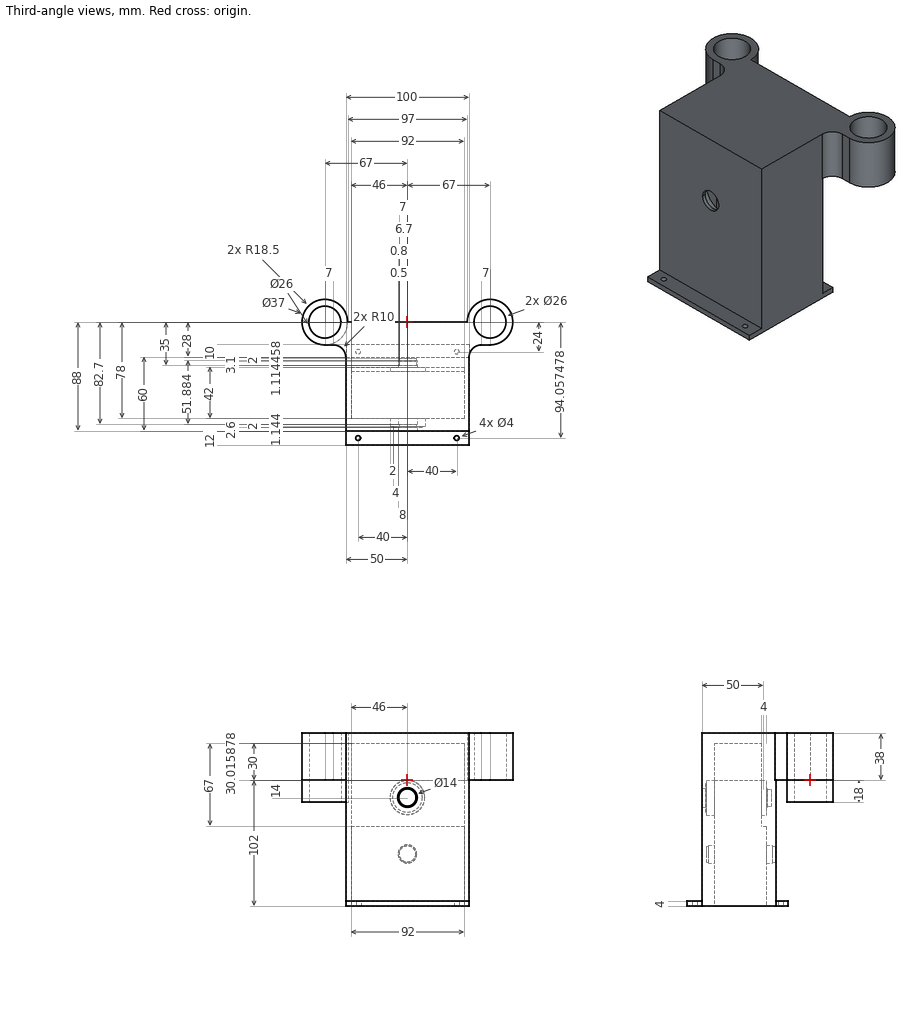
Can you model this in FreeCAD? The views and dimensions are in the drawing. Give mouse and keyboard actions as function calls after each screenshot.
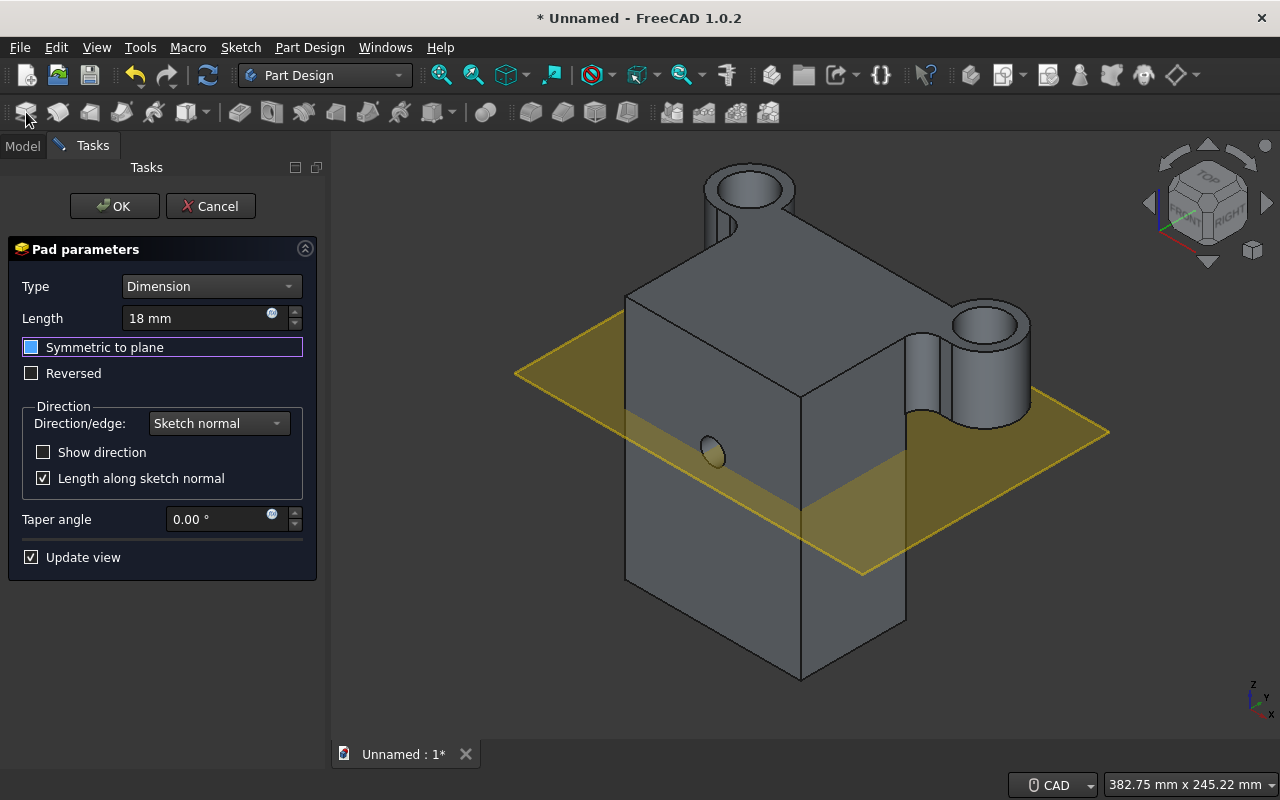
click(115, 206)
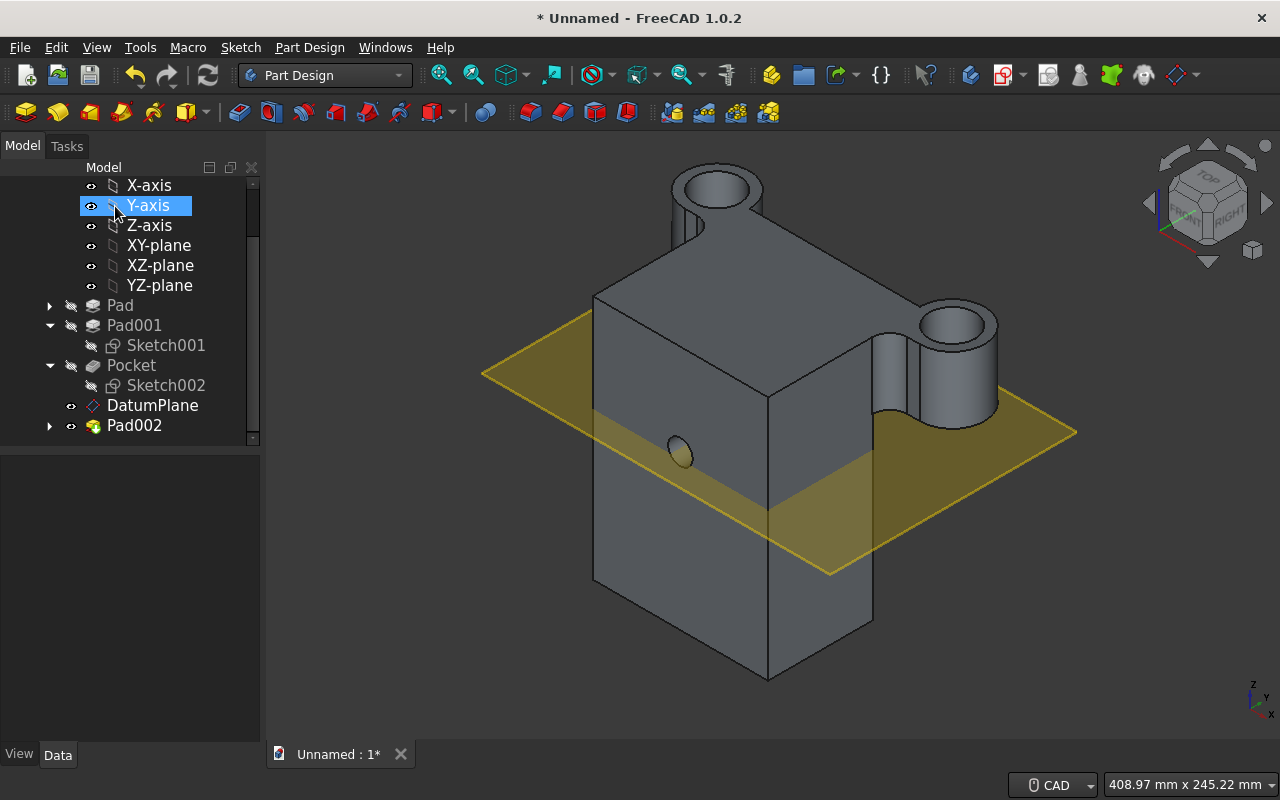
click(116, 406)
key(space)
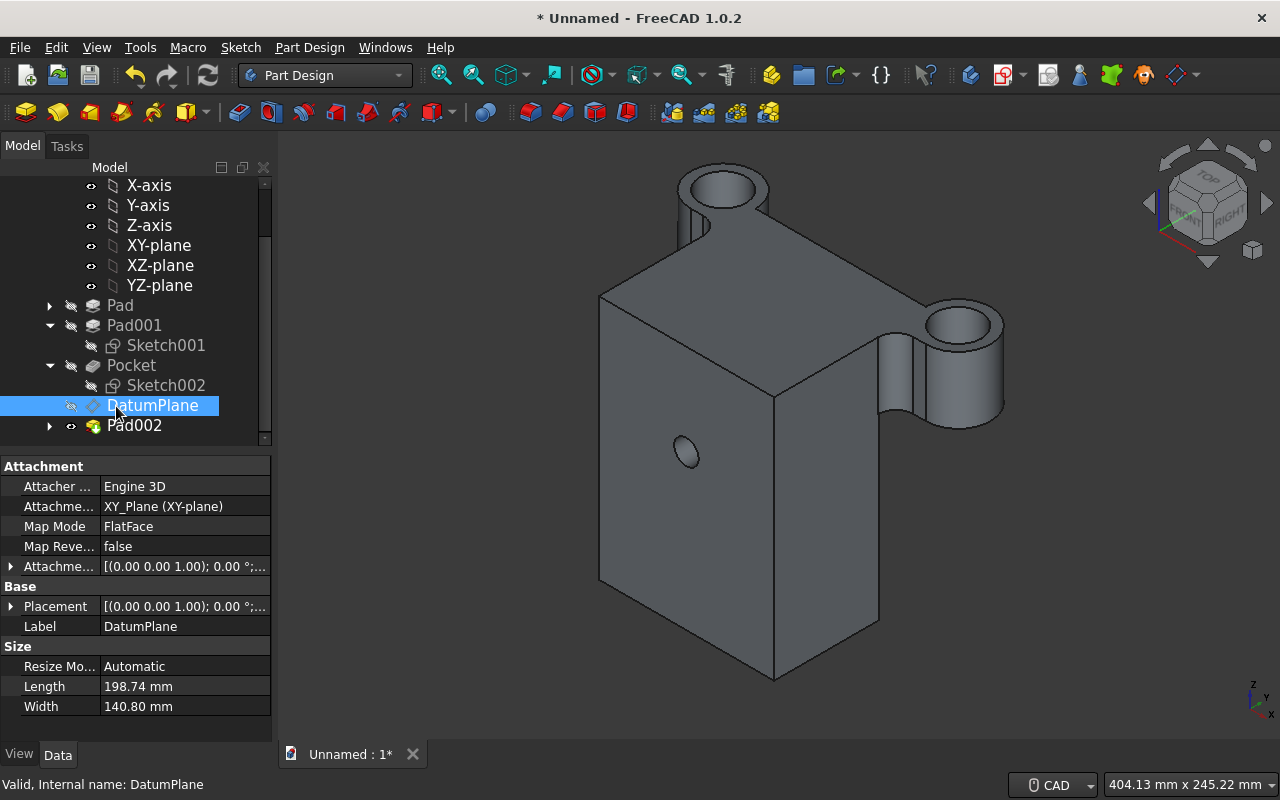
key(5)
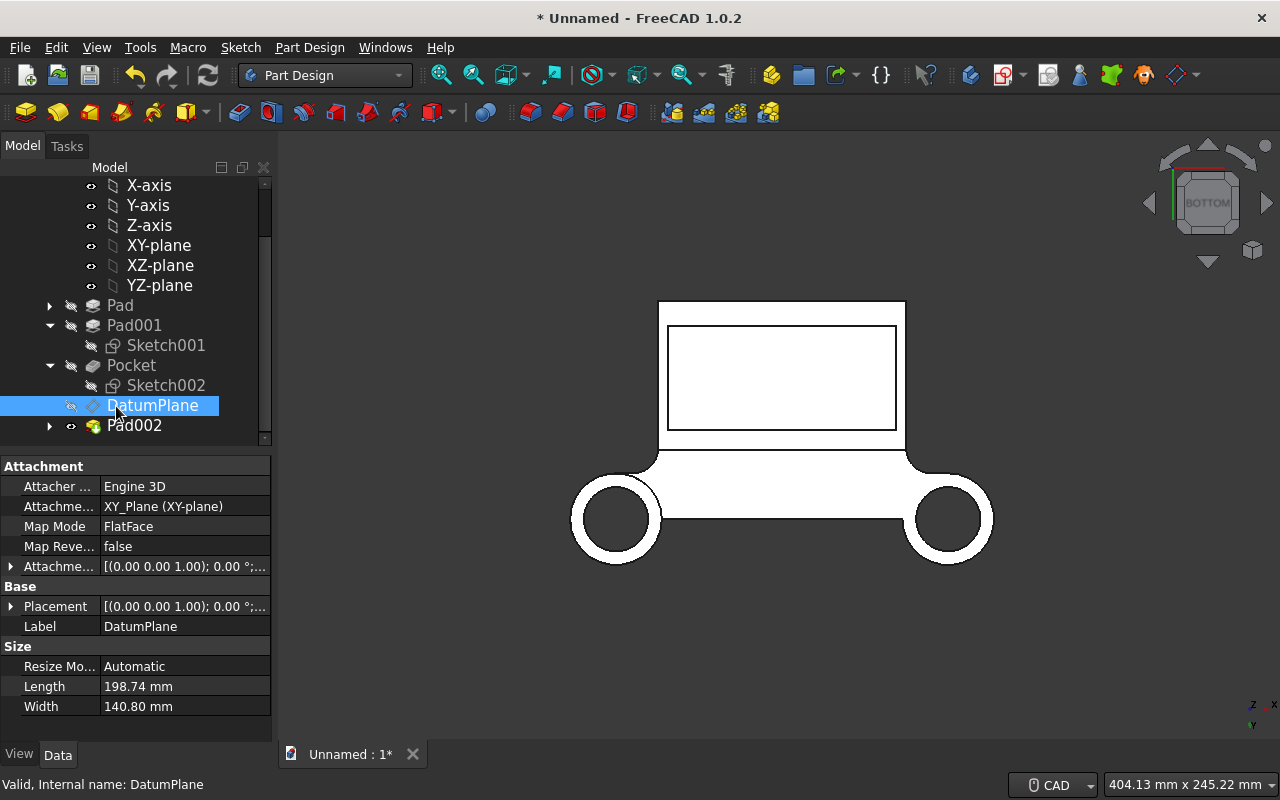
key(v)
key(f)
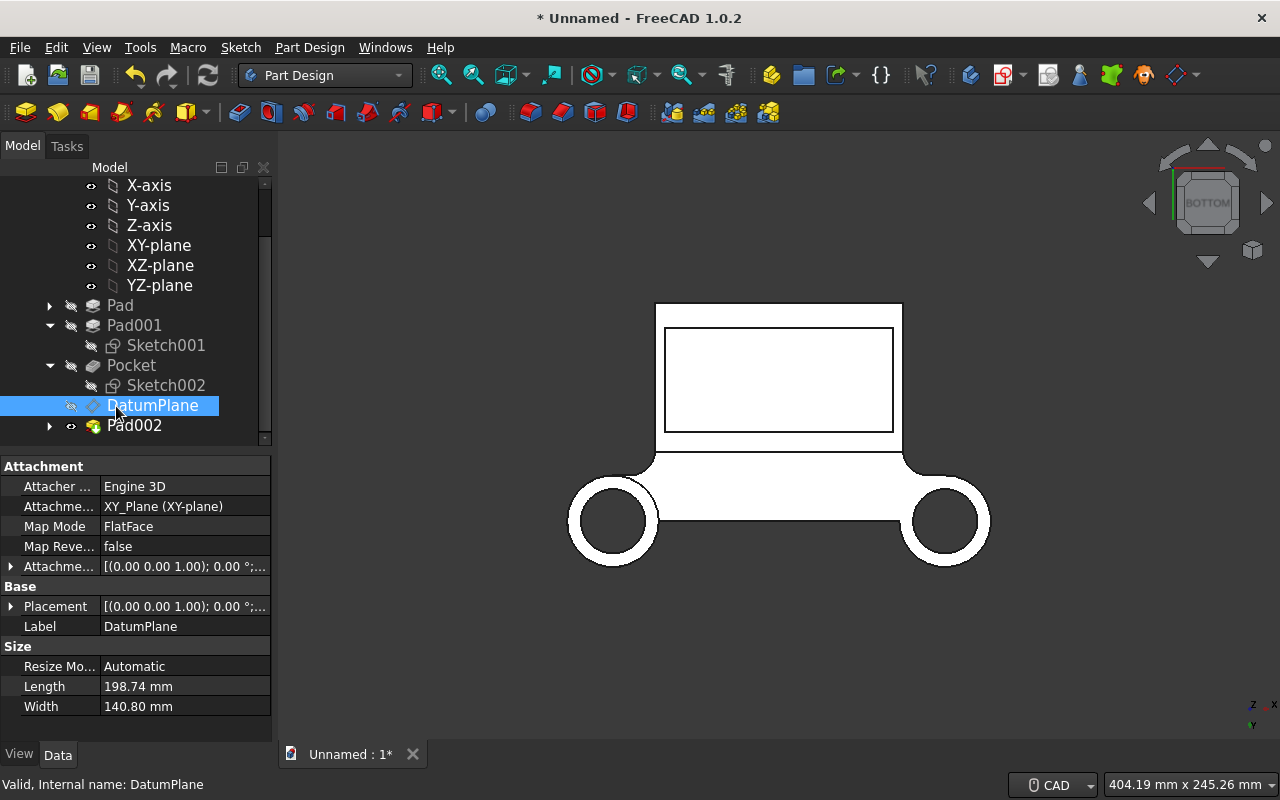
click(812, 379)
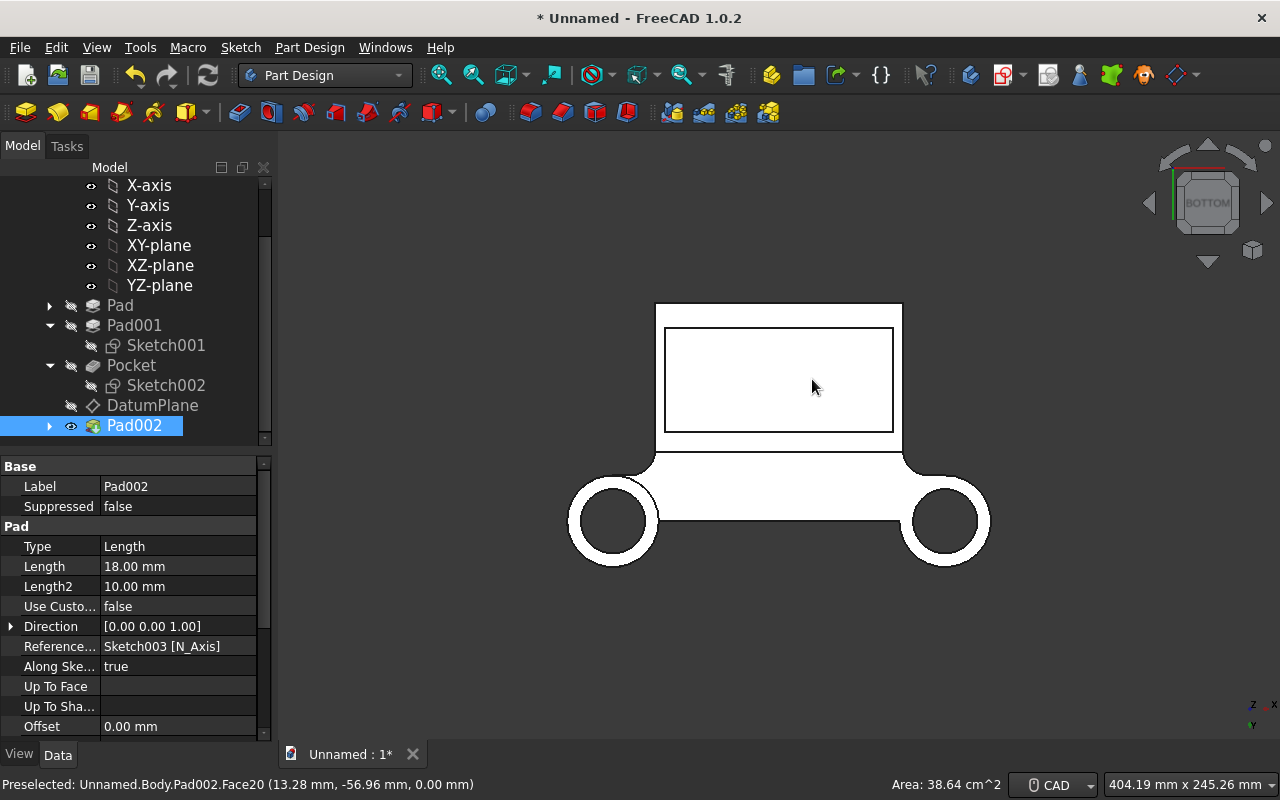
click(1004, 76)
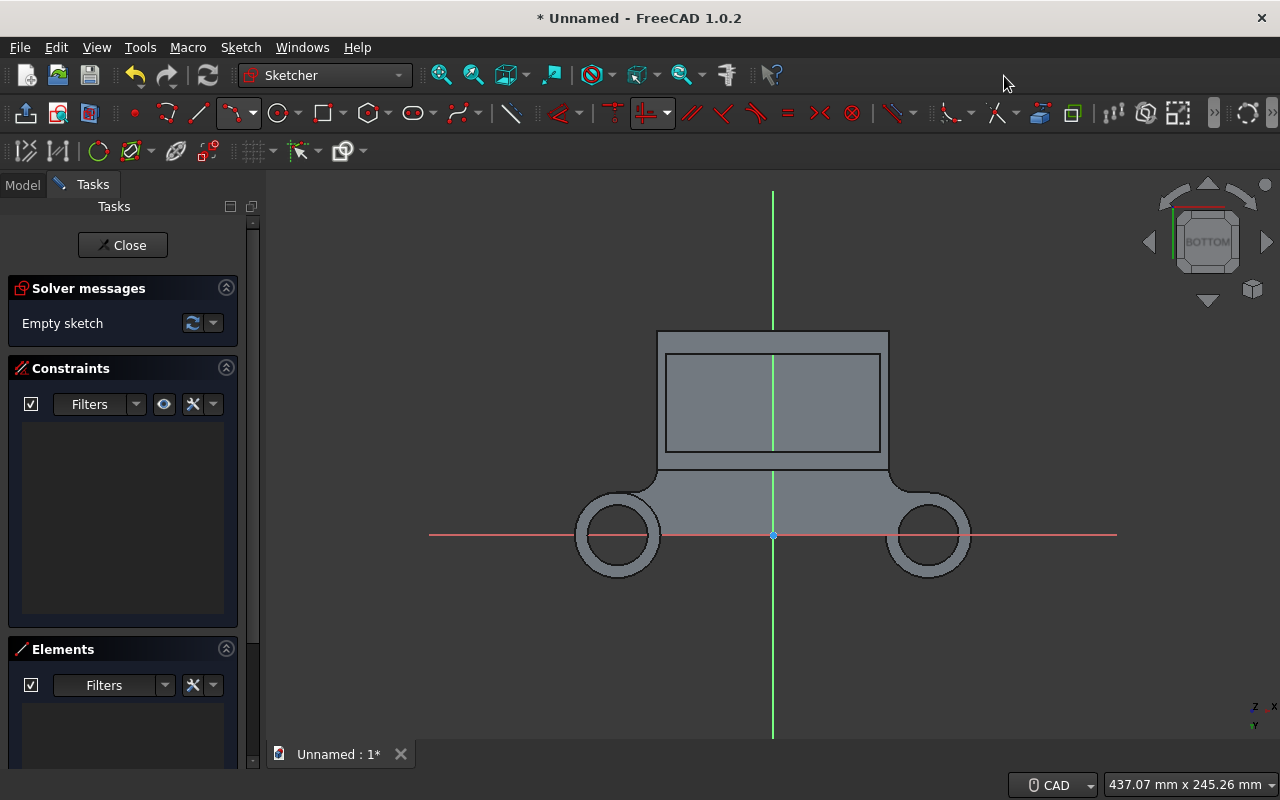
key(q)
key(s)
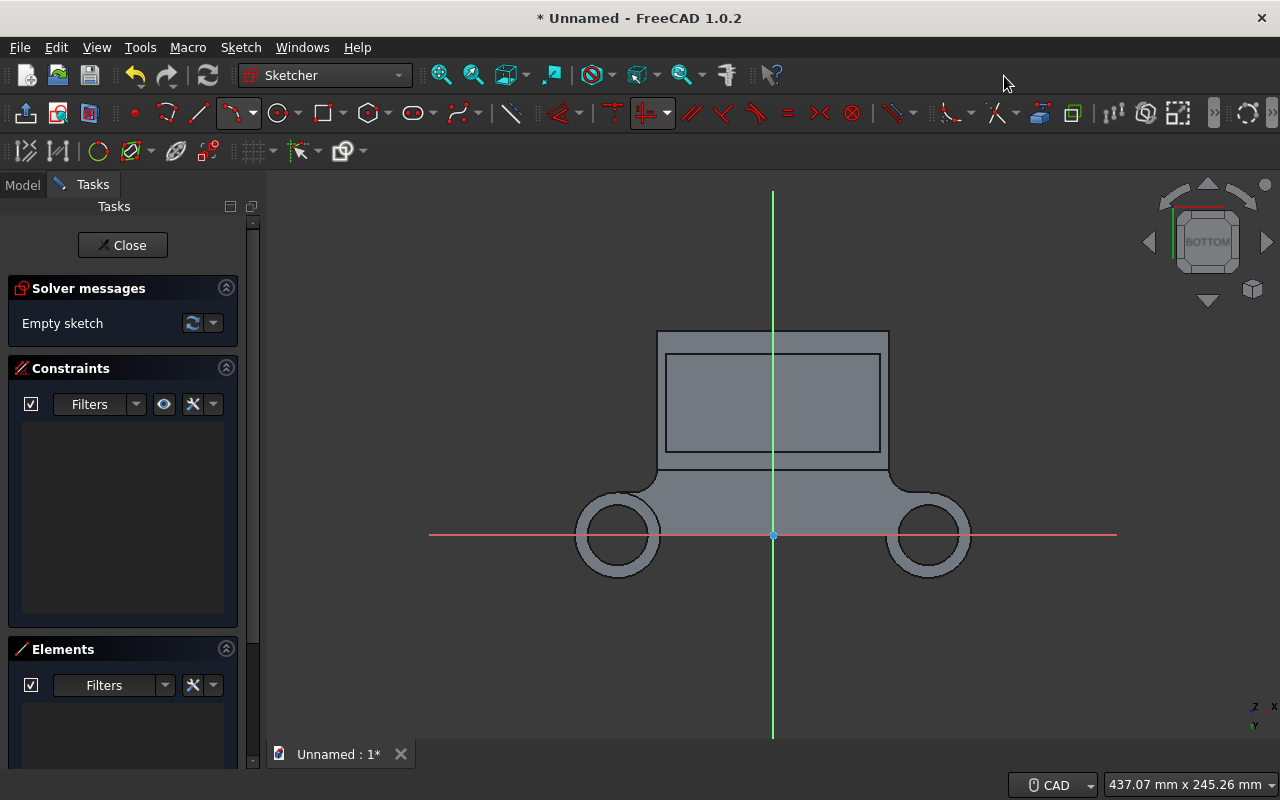
scroll(856, 433, up, 3)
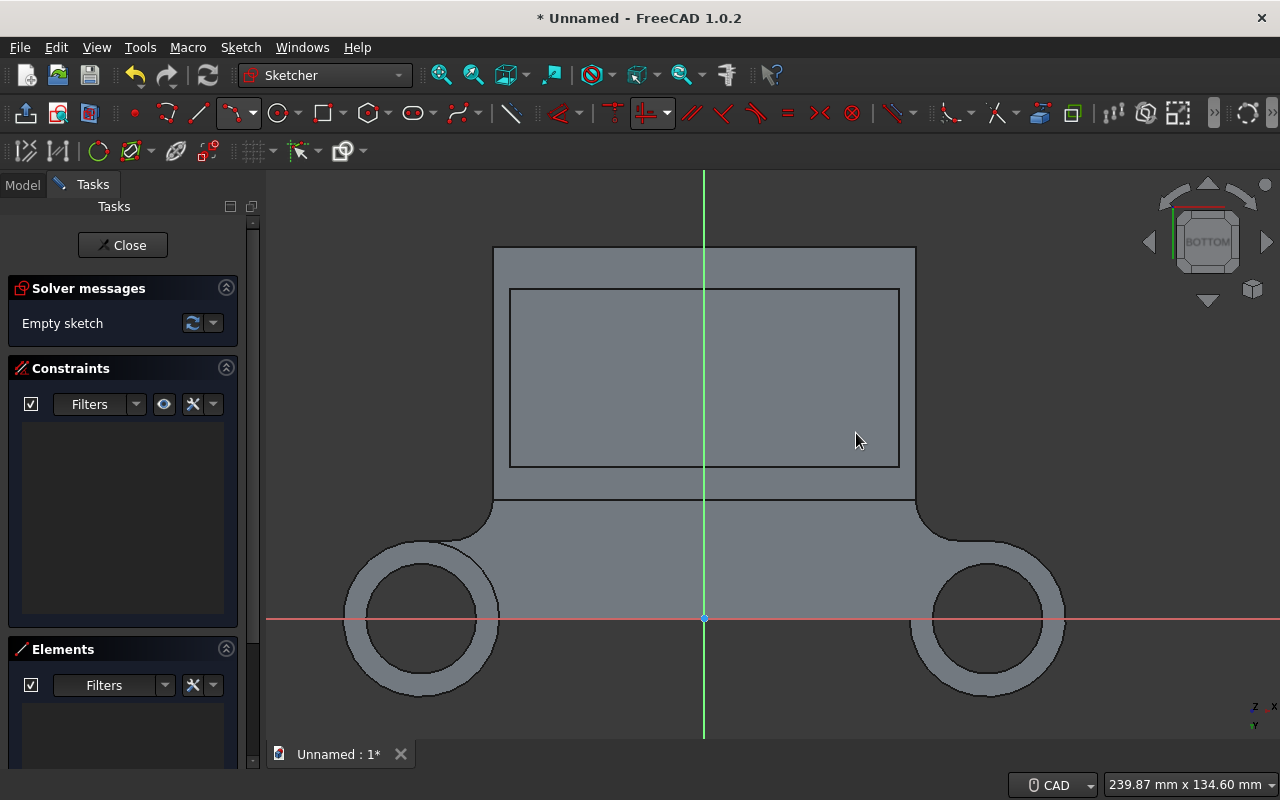
key(g)
key(r)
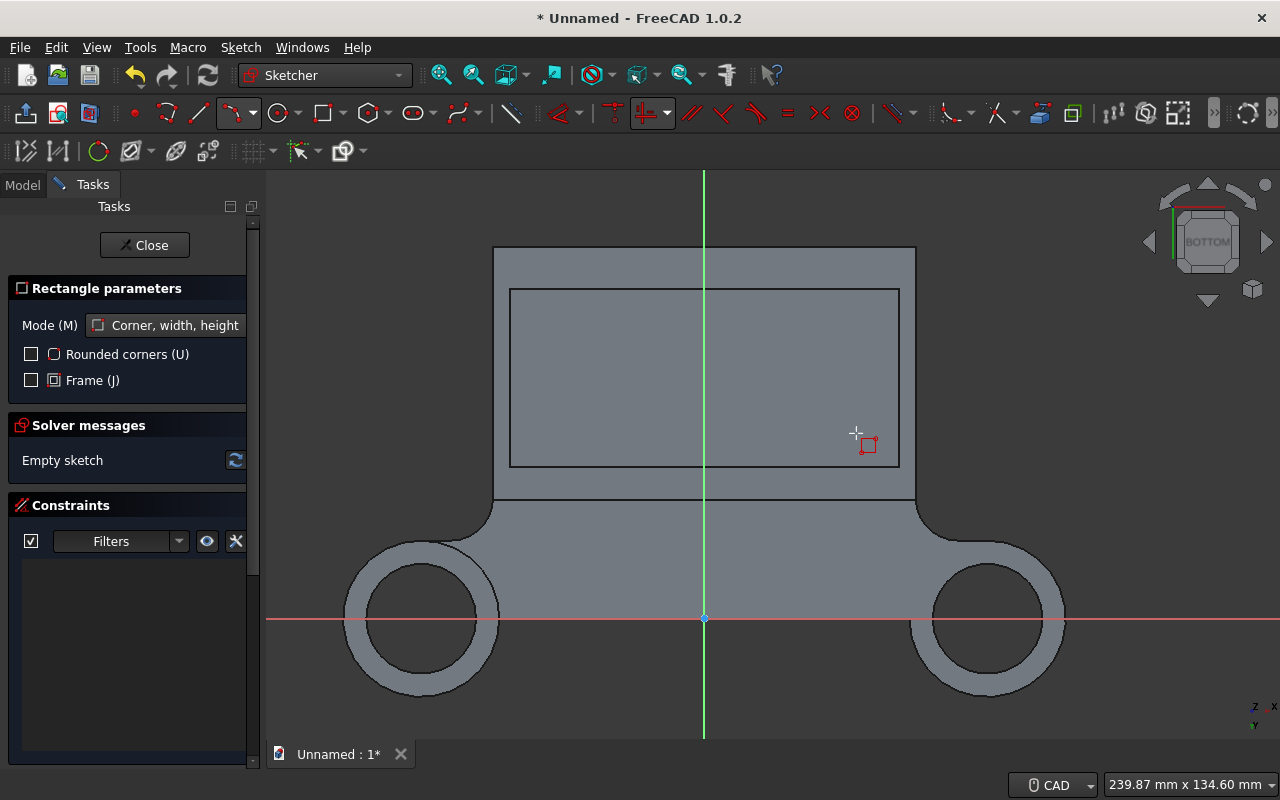
click(510, 289)
click(899, 467)
key(Escape)